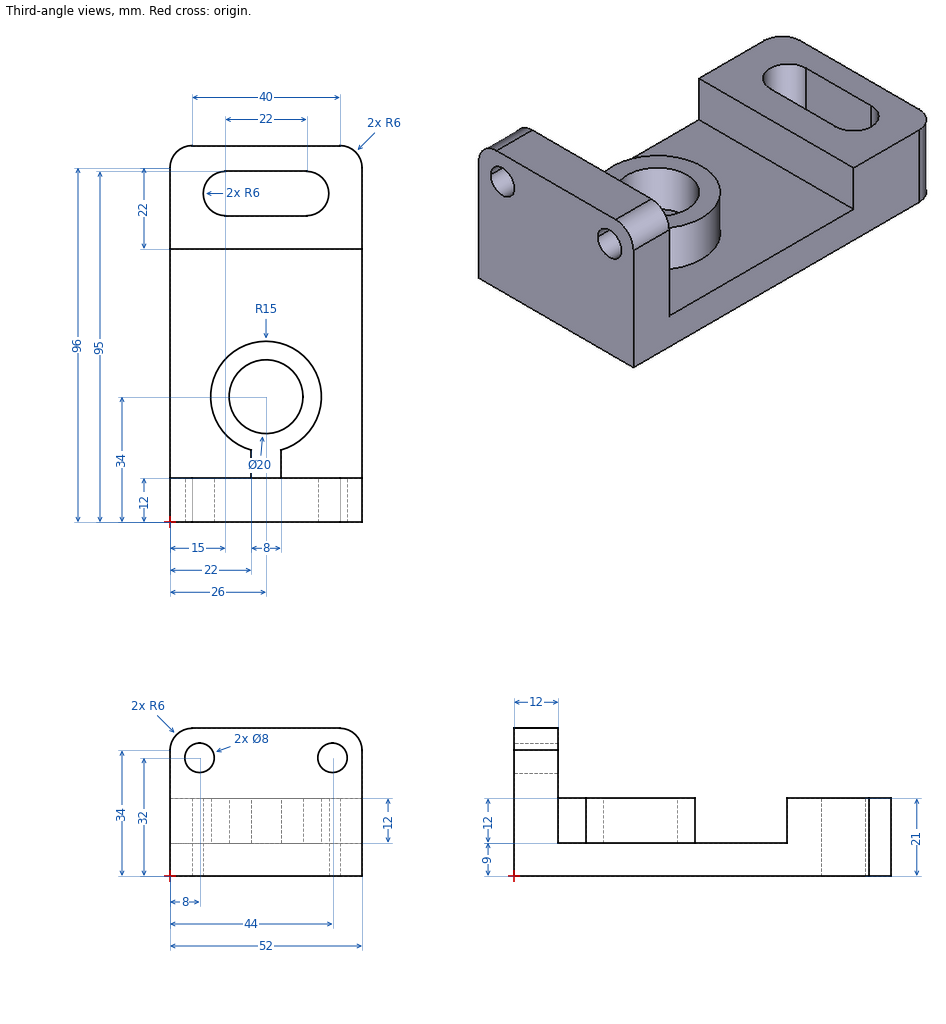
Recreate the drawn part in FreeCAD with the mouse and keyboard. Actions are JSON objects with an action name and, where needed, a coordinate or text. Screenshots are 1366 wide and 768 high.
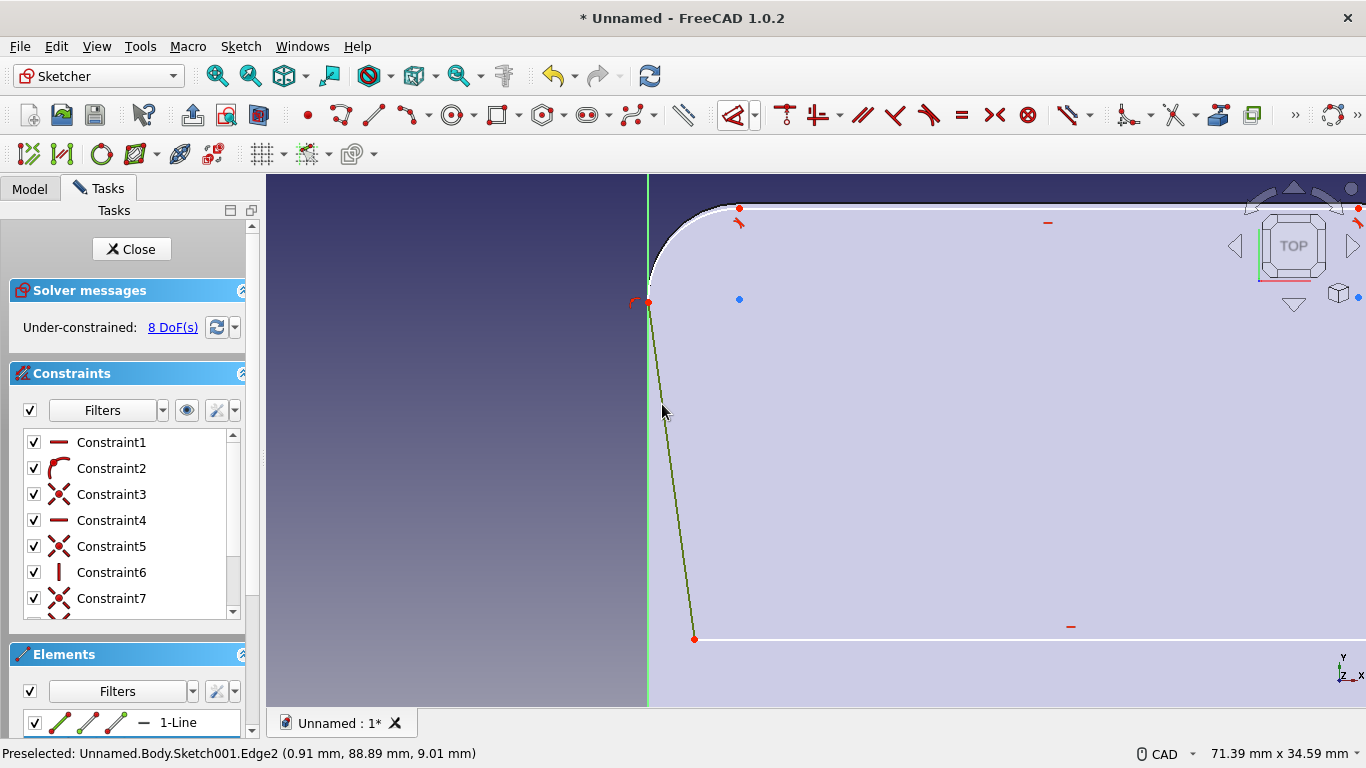
{"action": "scroll", "coordinate": [671, 302], "scroll_direction": "down", "scroll_amount": 8}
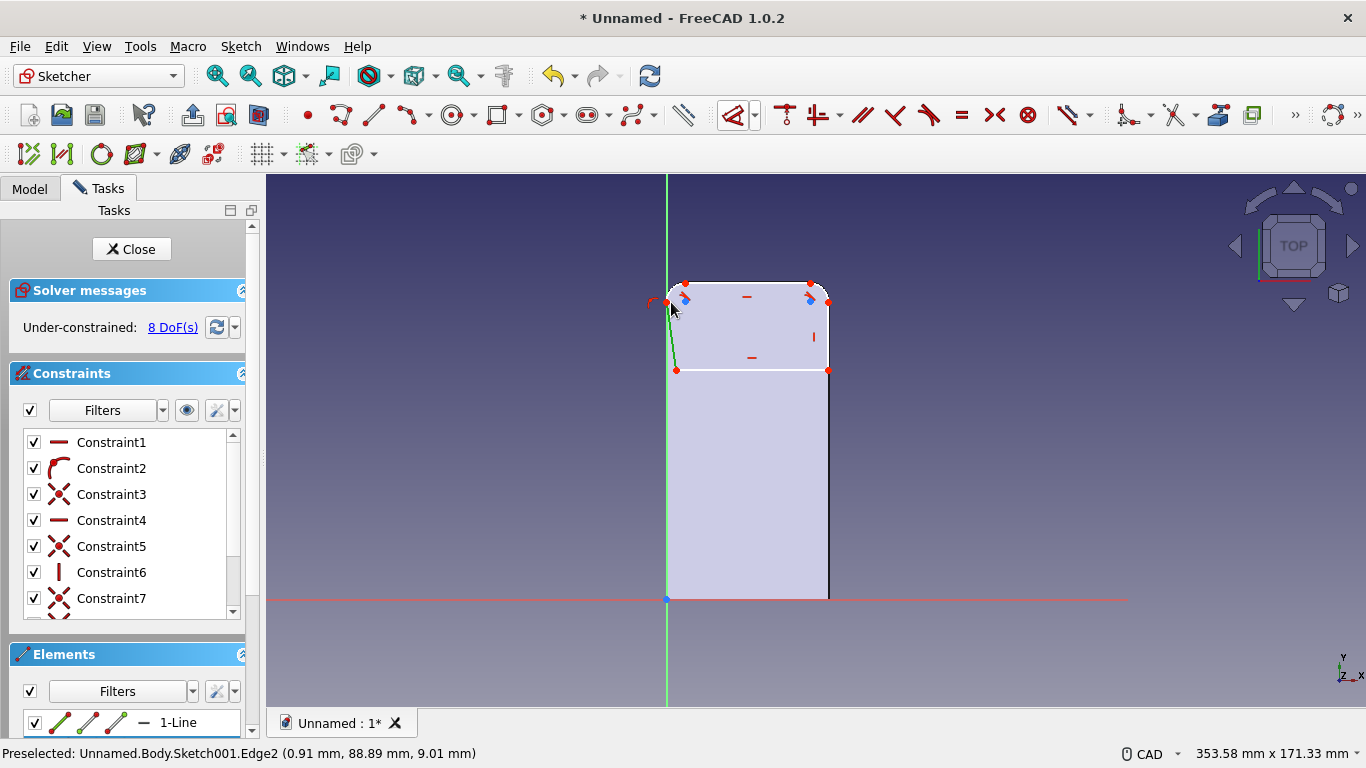
{"action": "scroll", "coordinate": [677, 285], "scroll_direction": "up", "scroll_amount": 3}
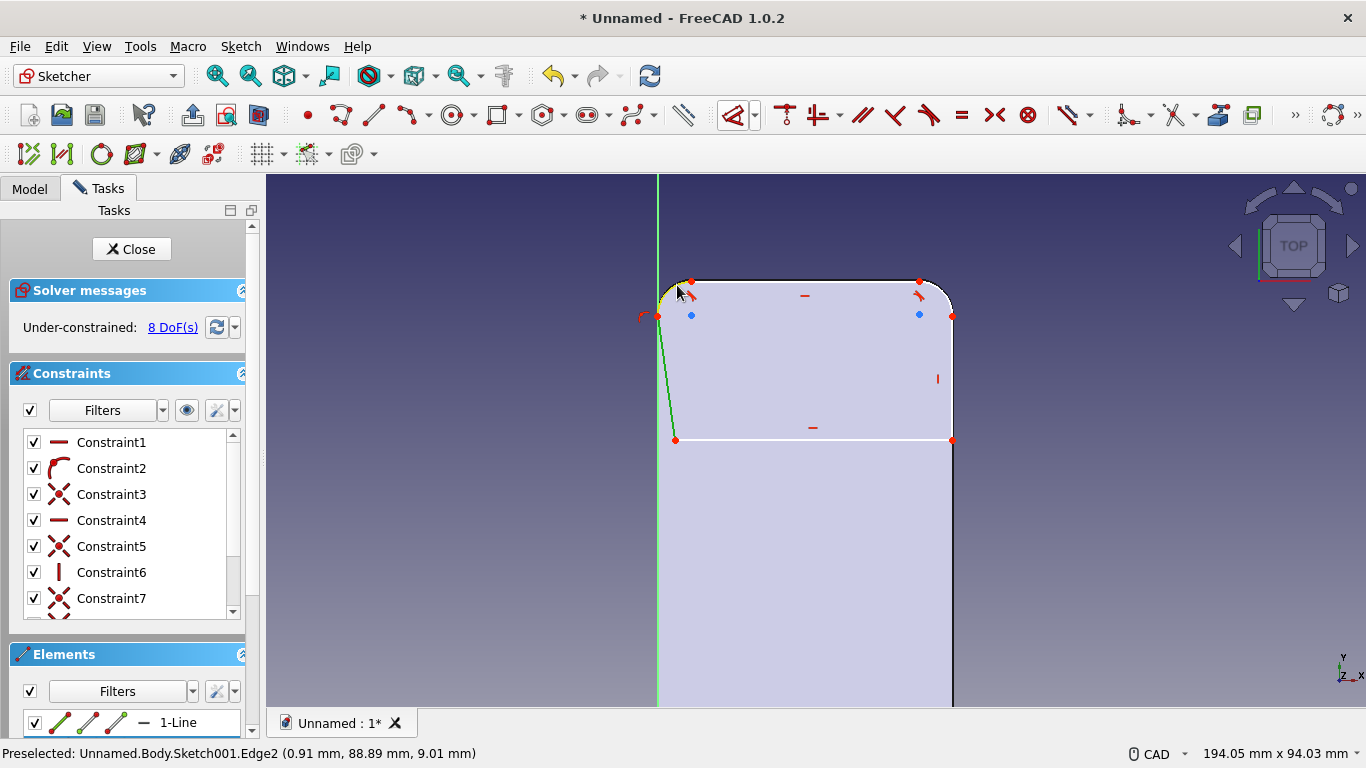
{"action": "left_click", "coordinate": [676, 286]}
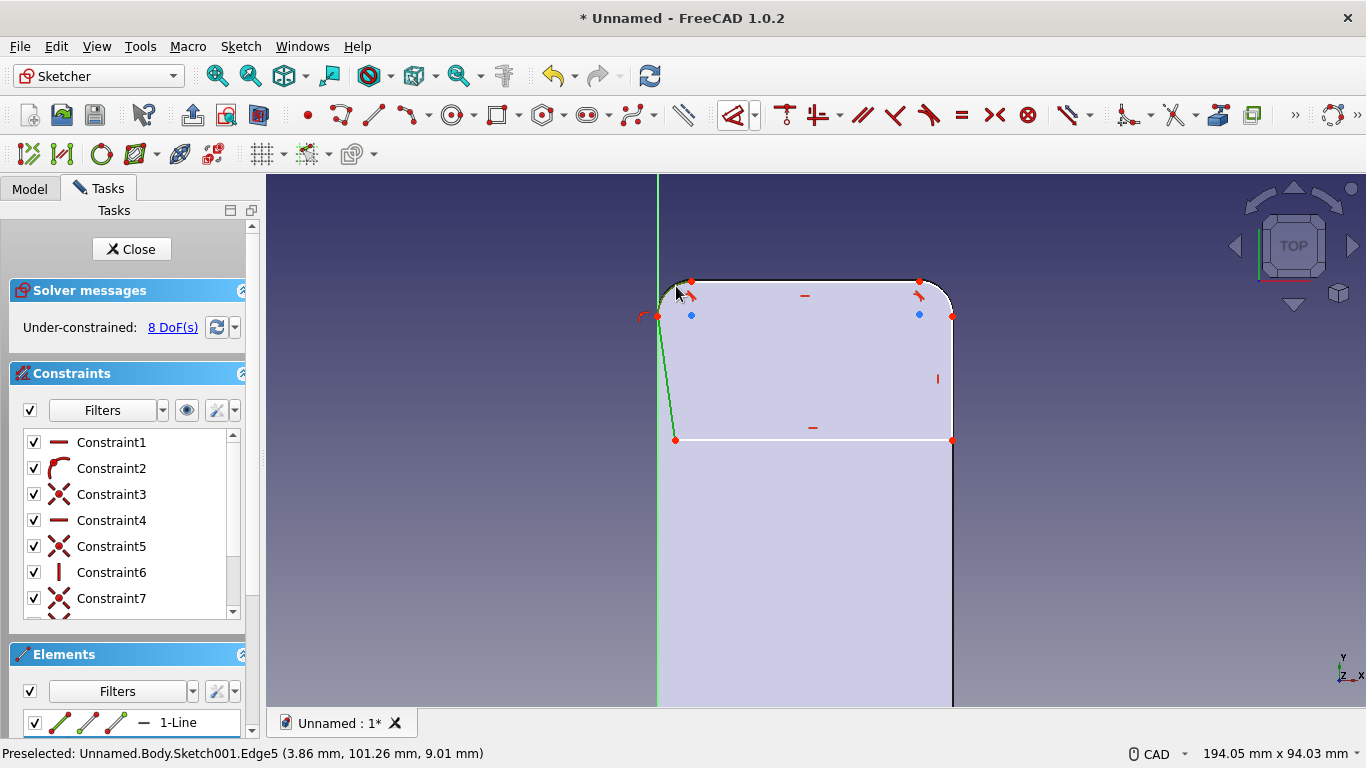
{"action": "left_click", "coordinate": [929, 116]}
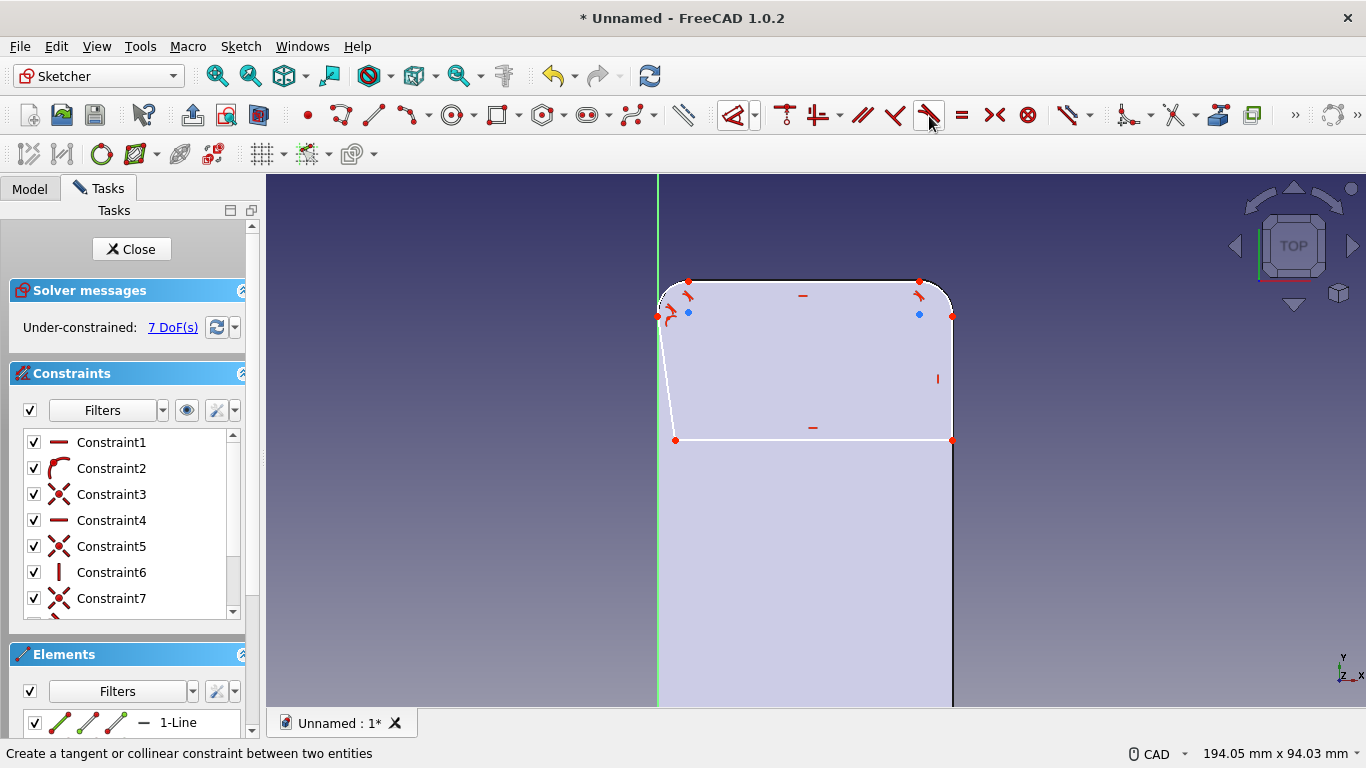
{"action": "left_click", "coordinate": [952, 403]}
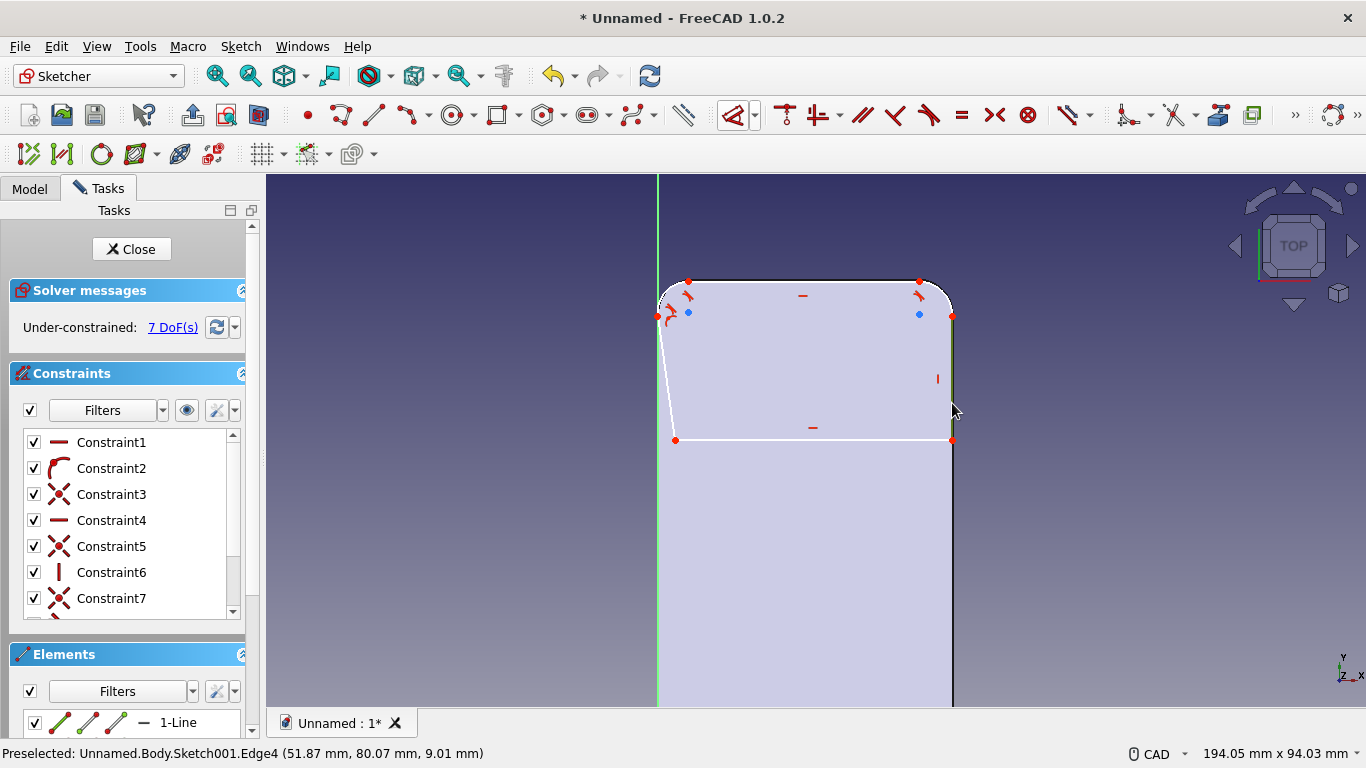
{"action": "left_click", "coordinate": [949, 301]}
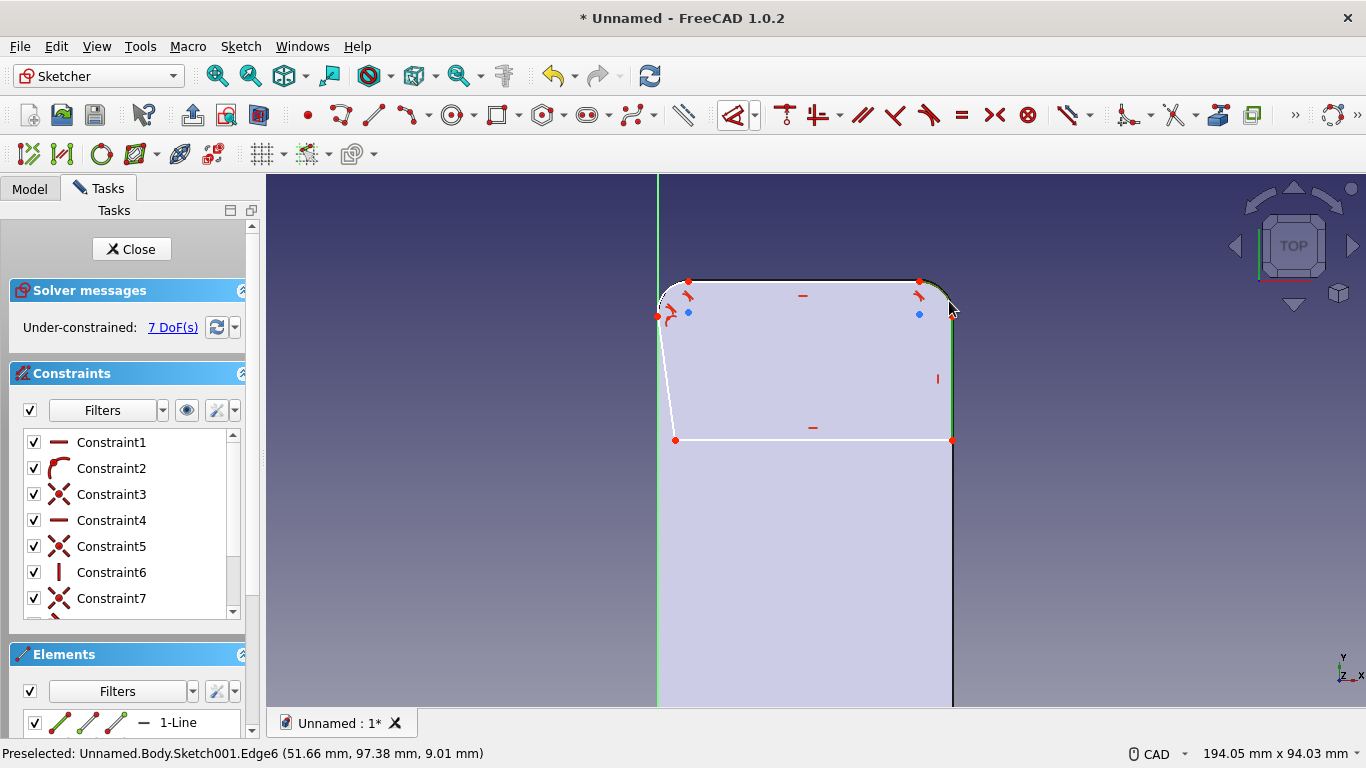
{"action": "left_click", "coordinate": [929, 116]}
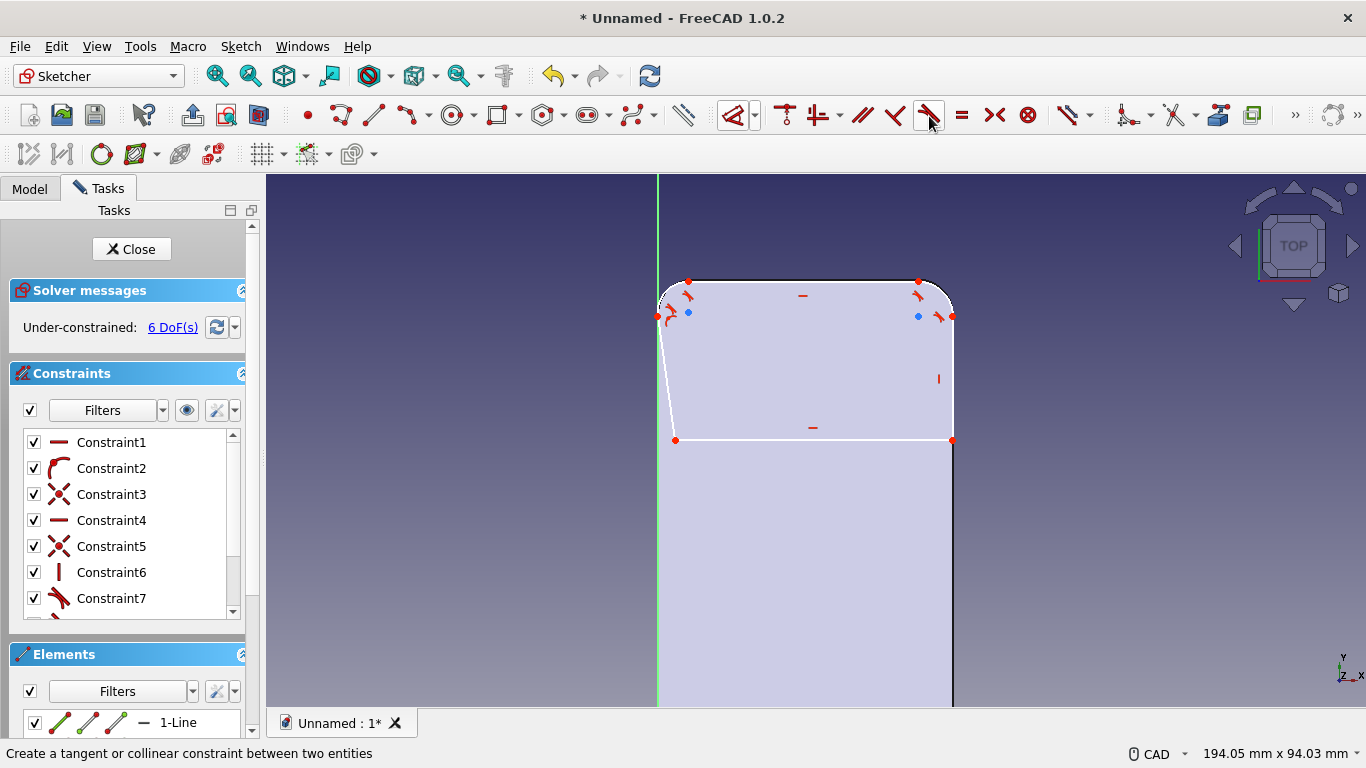
{"action": "left_click", "coordinate": [670, 403]}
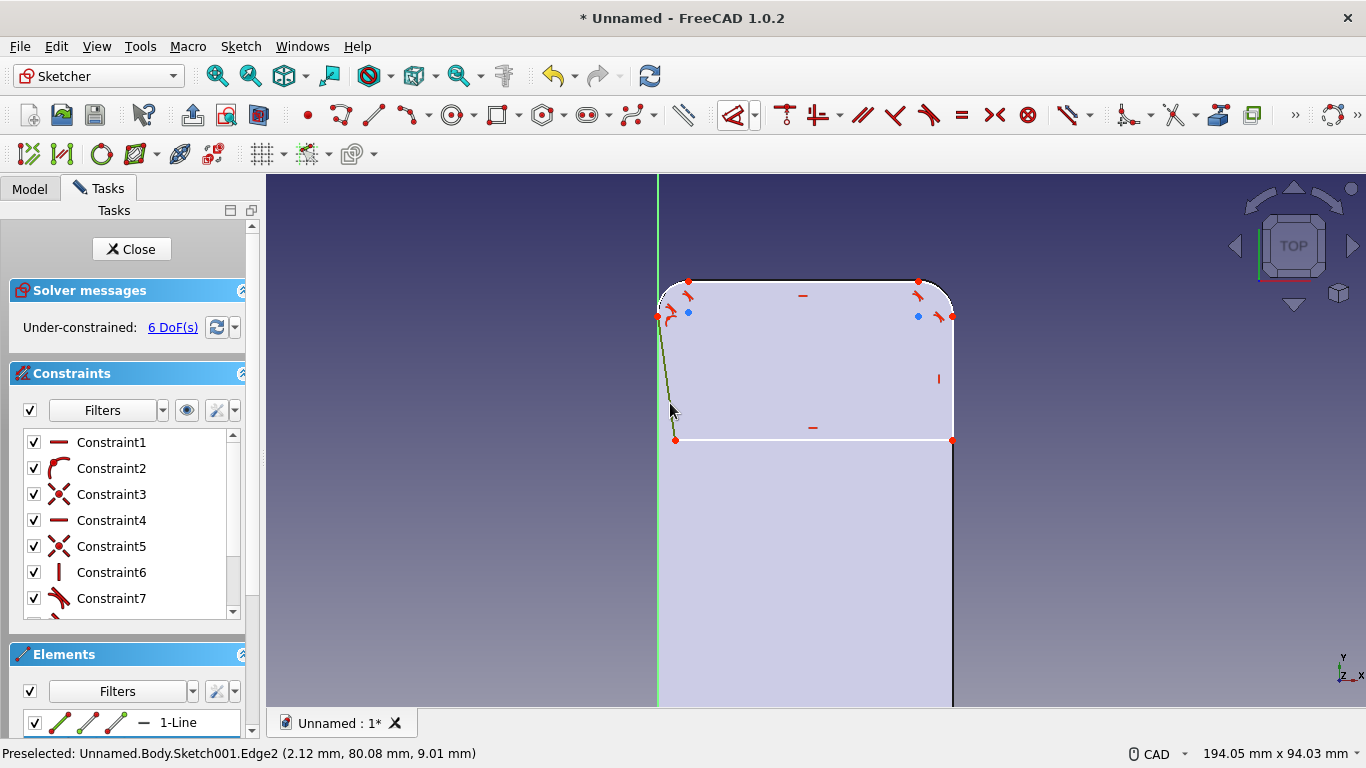
{"action": "left_click", "coordinate": [840, 116]}